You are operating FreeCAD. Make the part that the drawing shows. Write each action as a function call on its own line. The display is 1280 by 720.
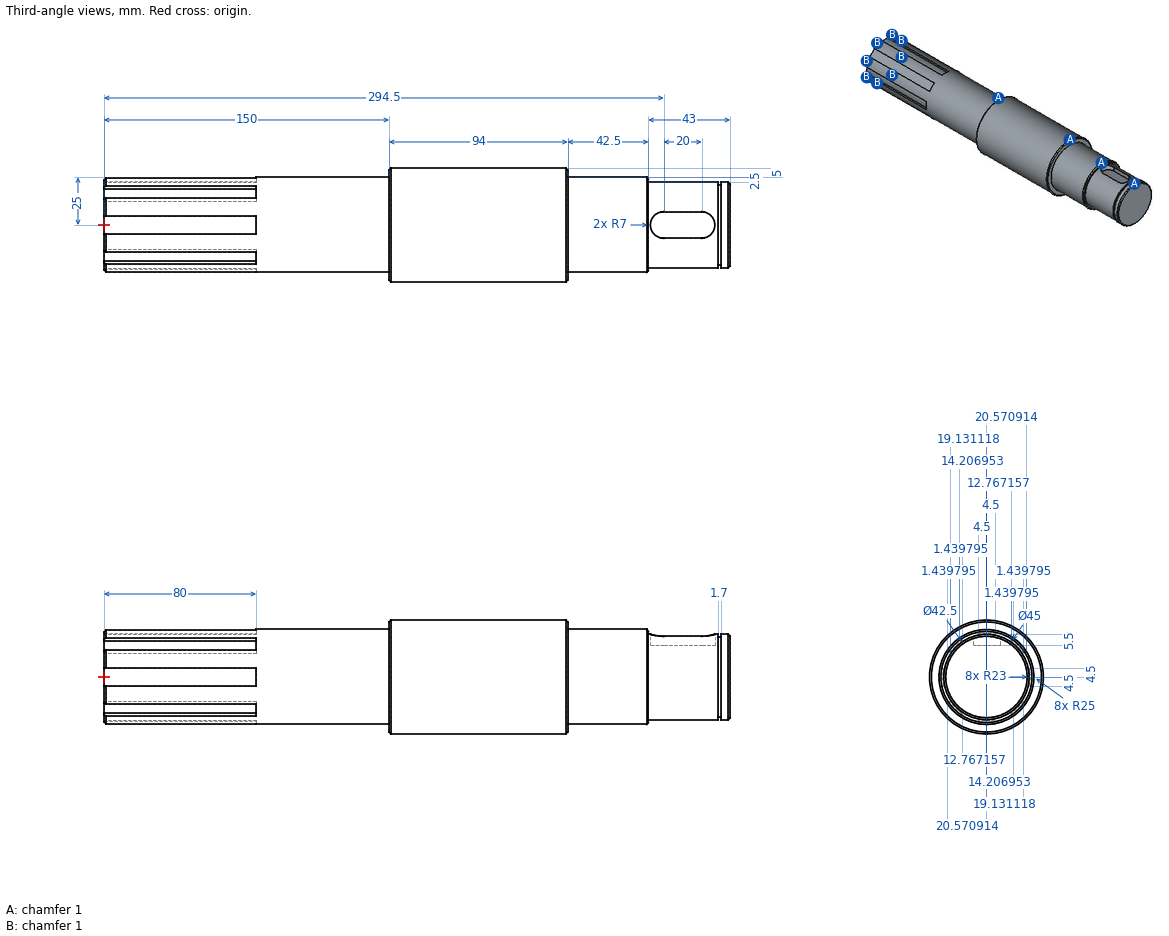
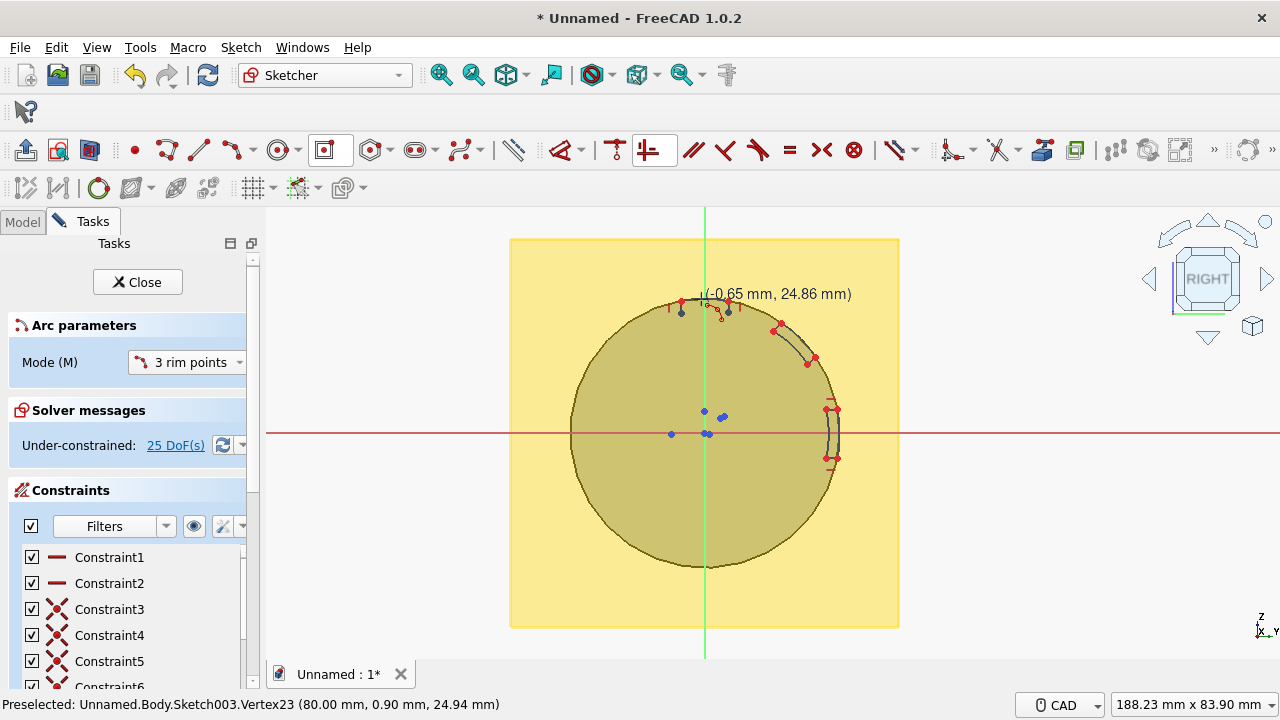
scroll(729, 312, up, 6)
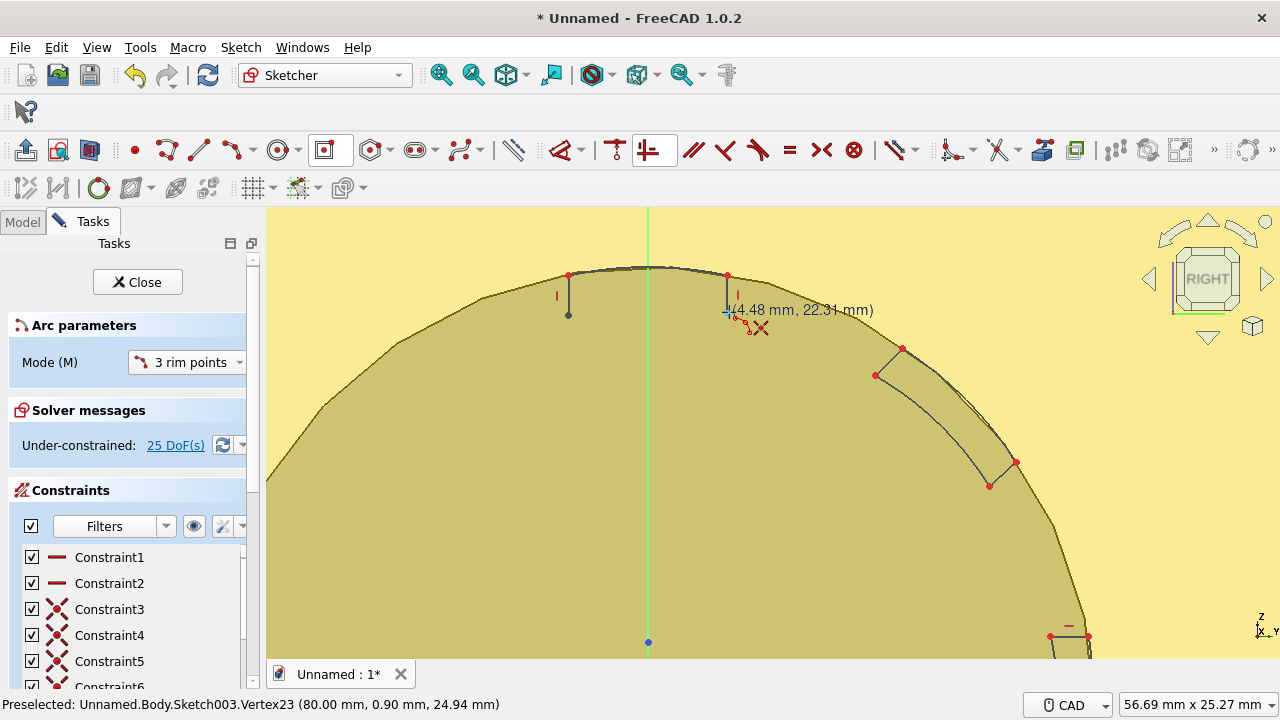
click(727, 313)
click(569, 315)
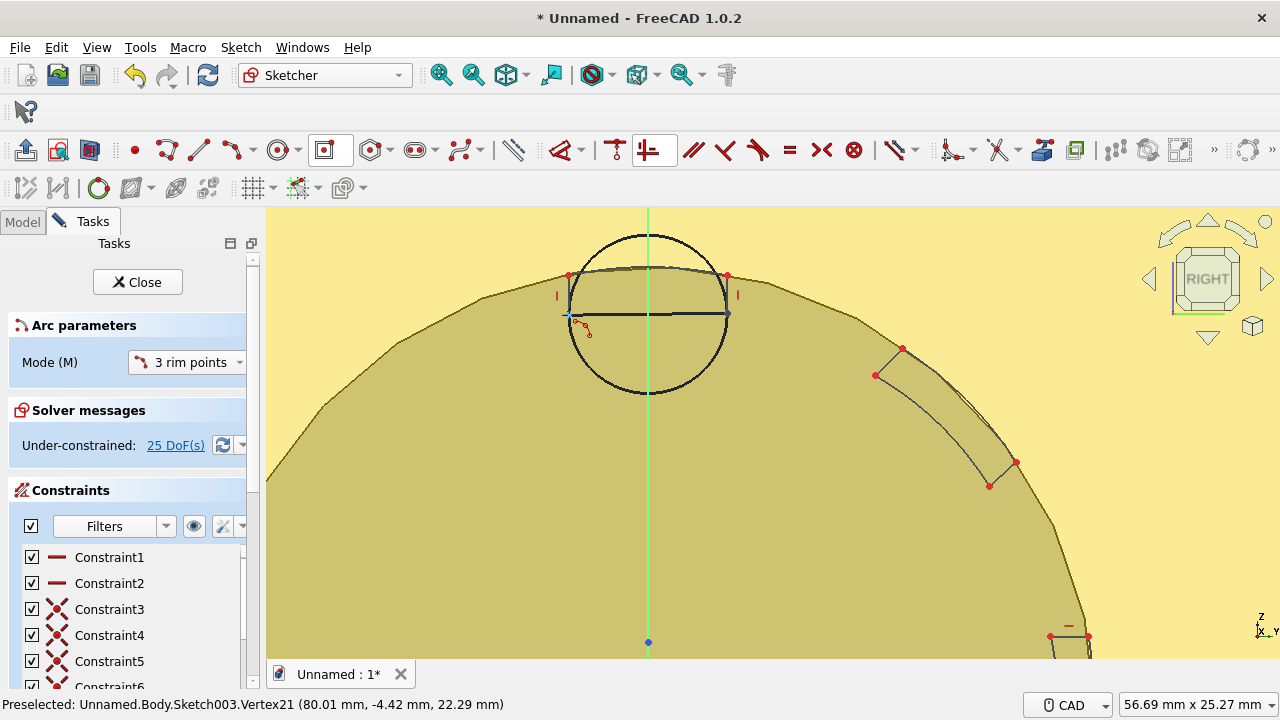
scroll(664, 303, up, 4)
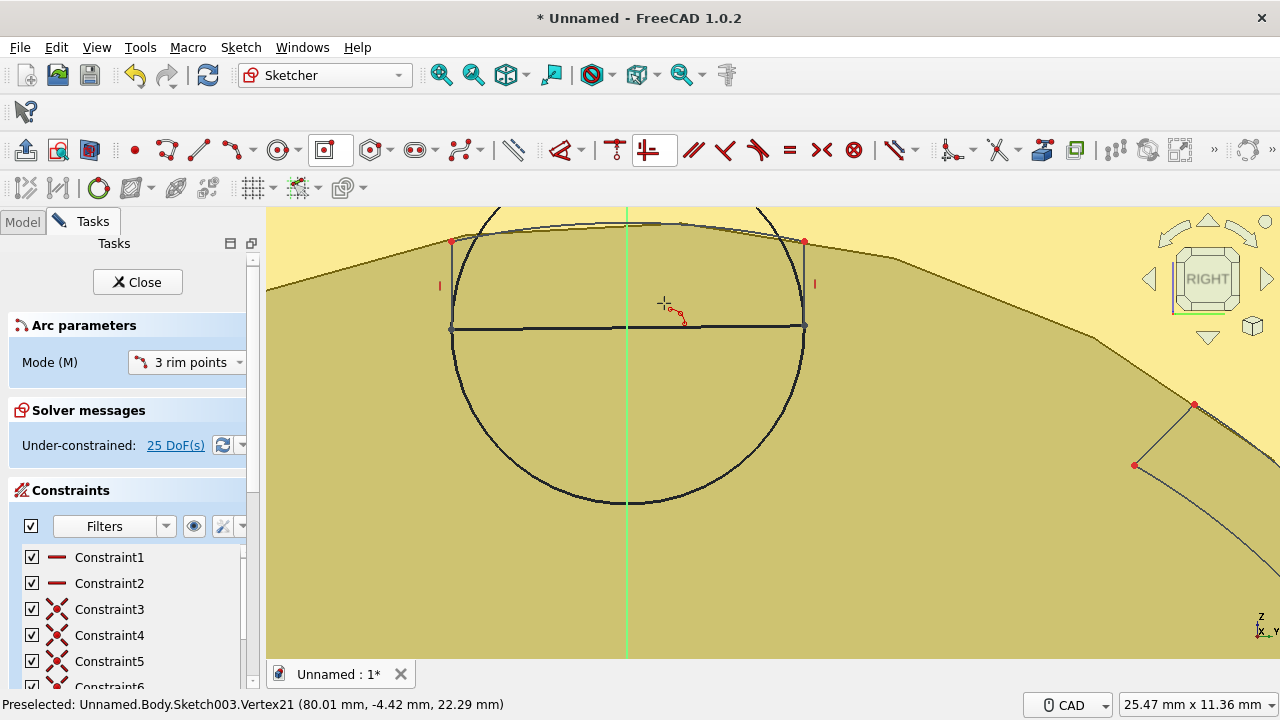
click(664, 302)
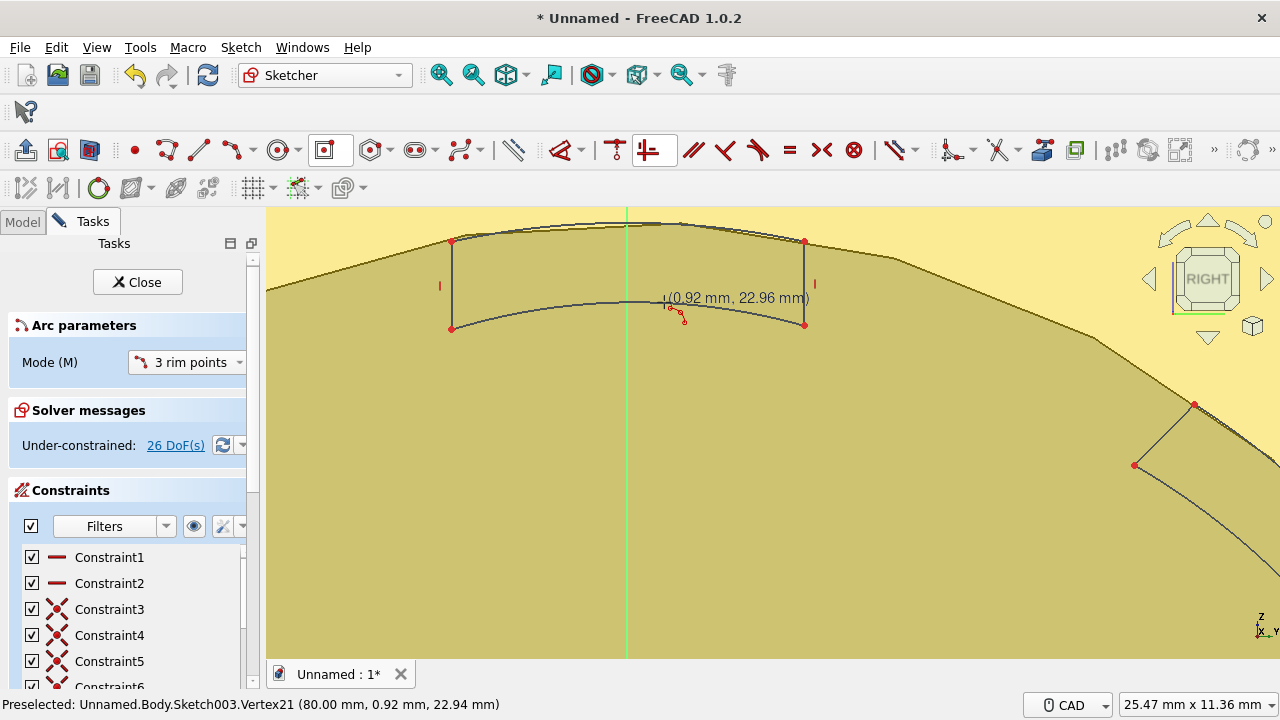
click(200, 150)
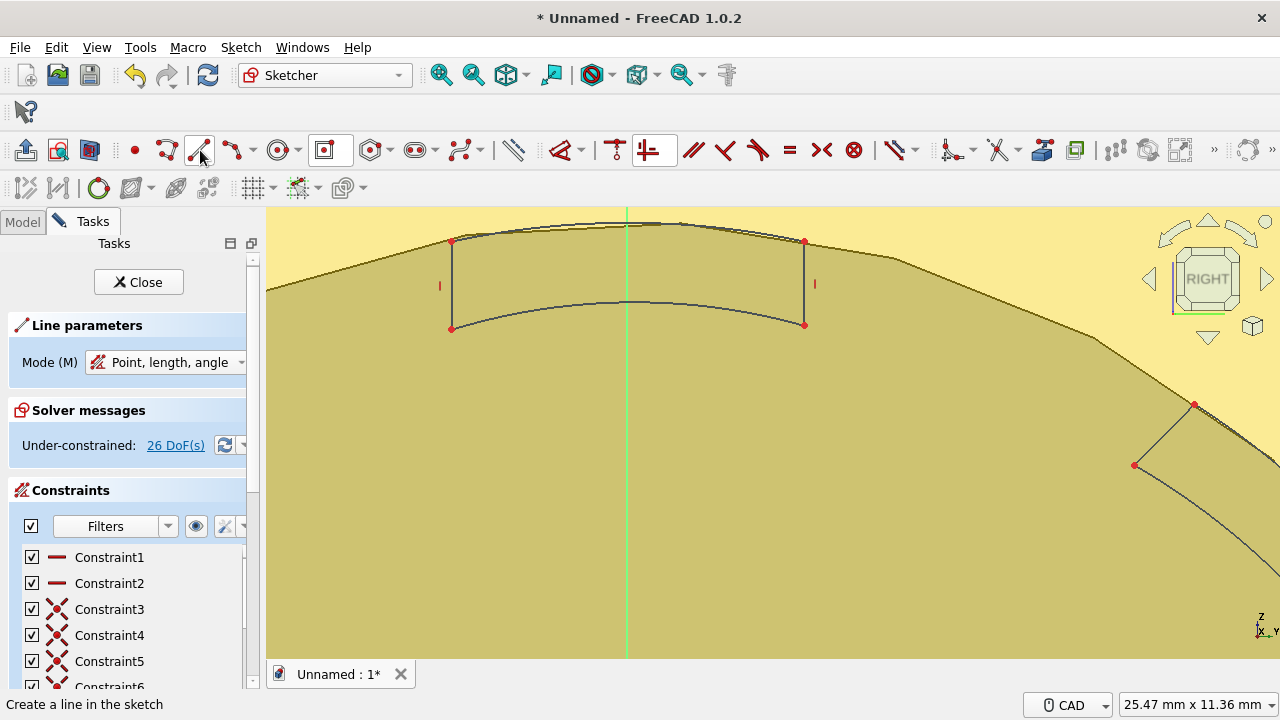
scroll(717, 310, down, 10)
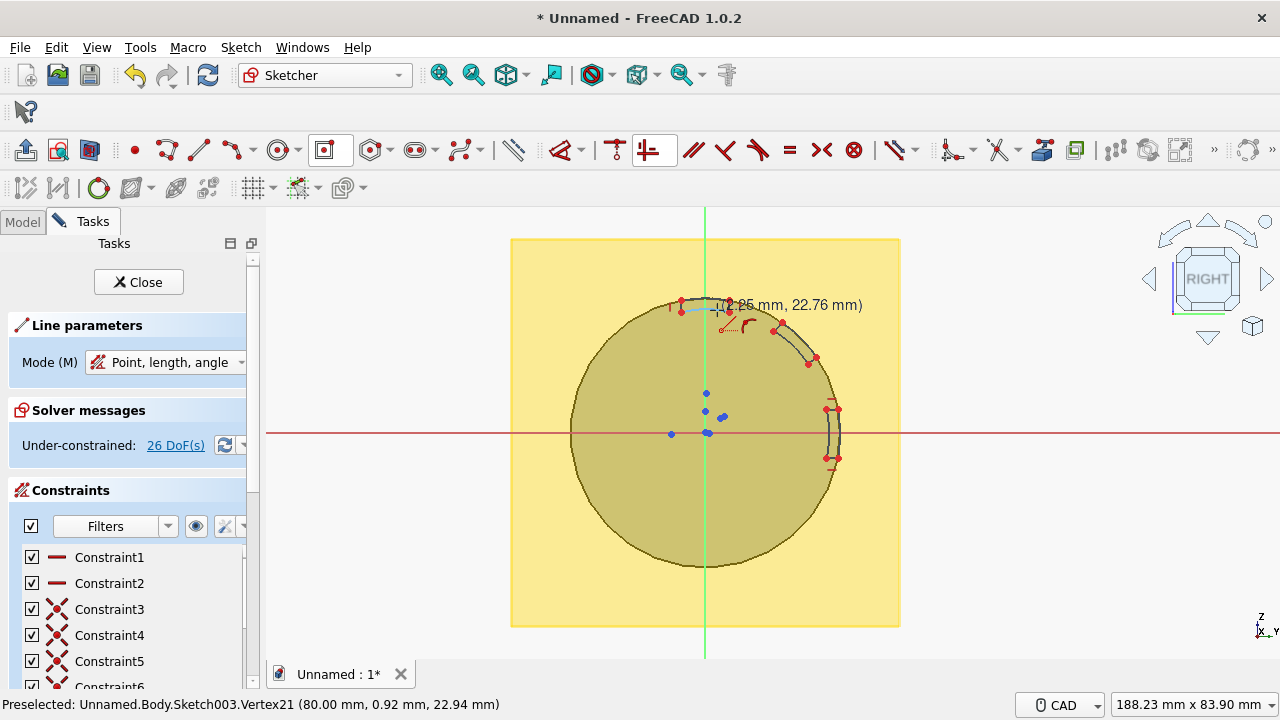
click(602, 364)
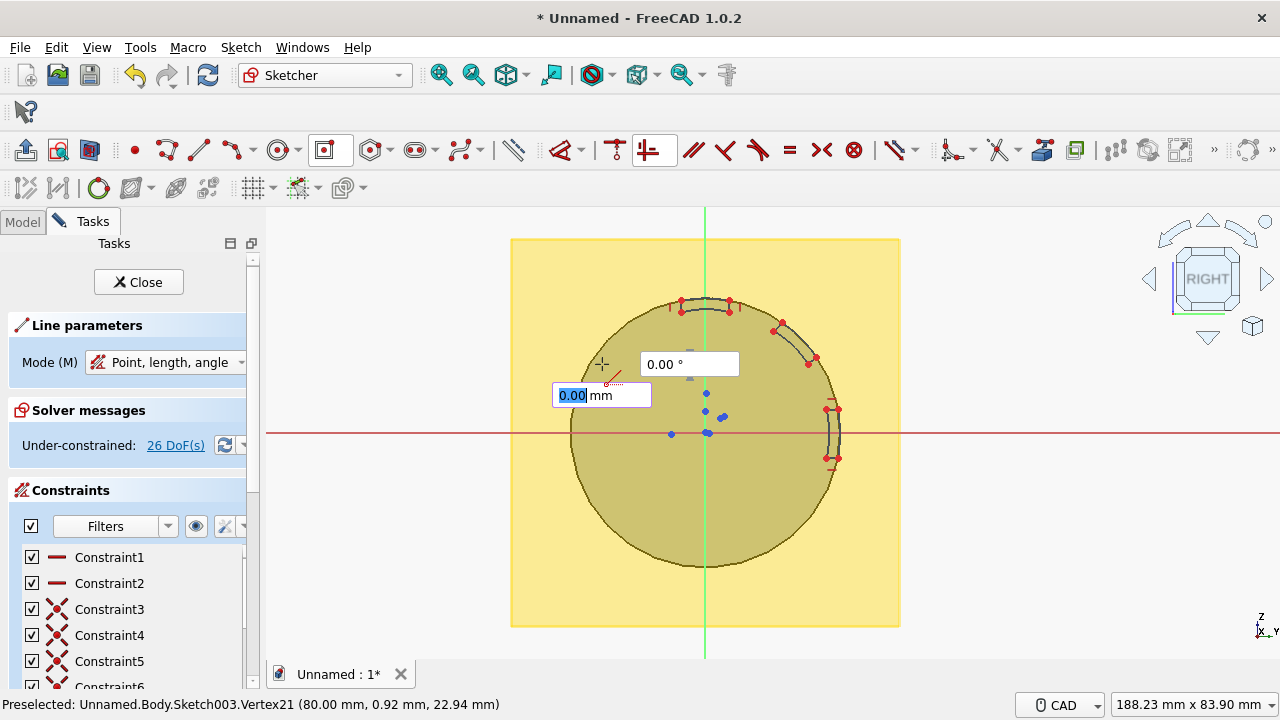
scroll(594, 356, up, 2)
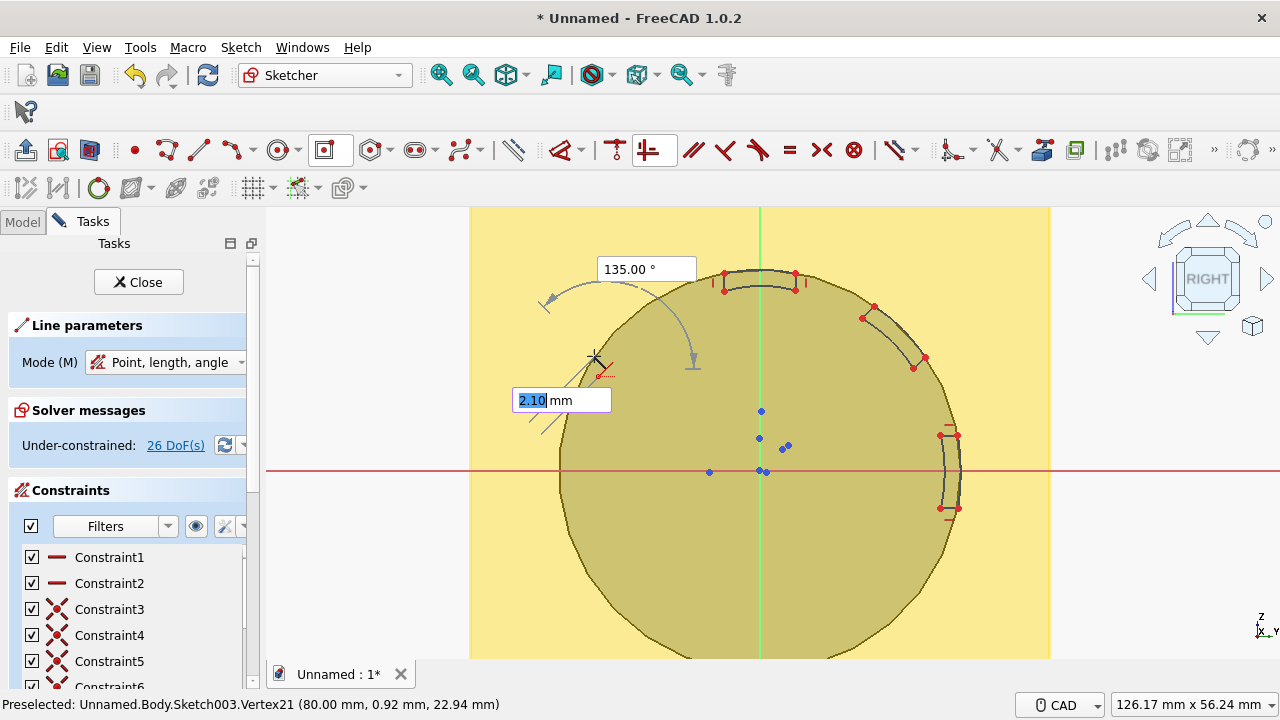
click(595, 356)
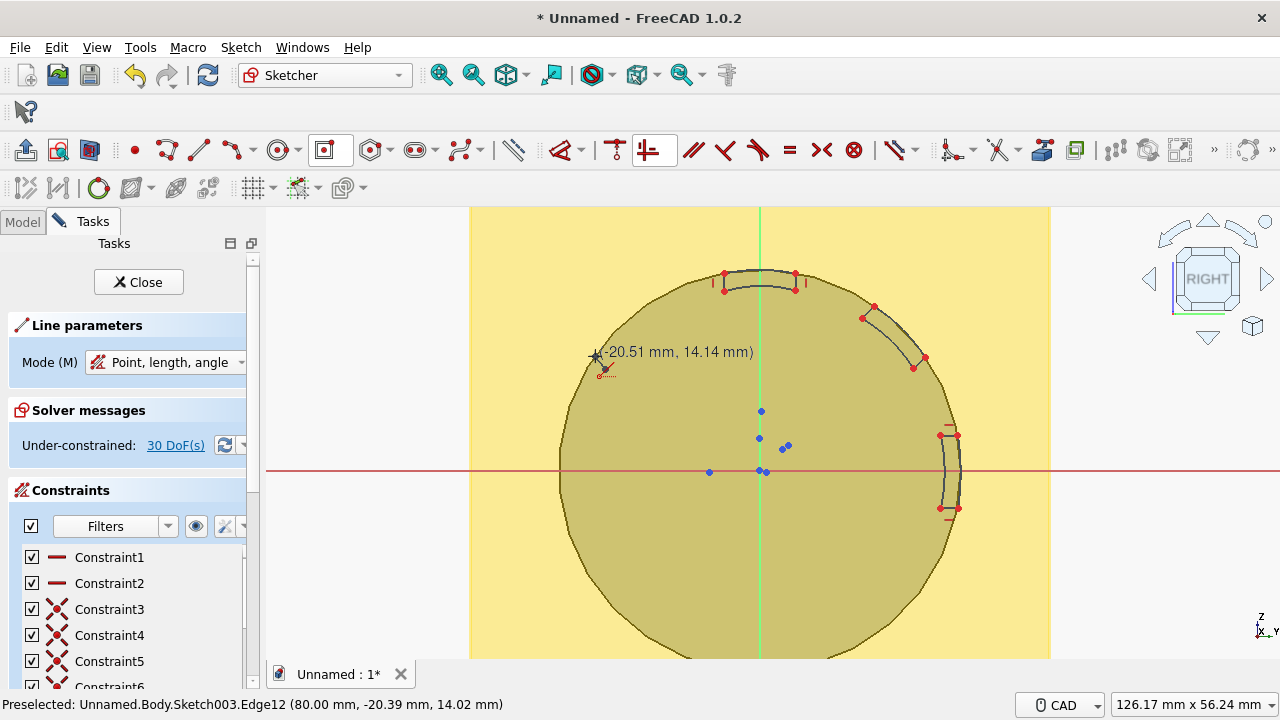
click(646, 305)
click(657, 317)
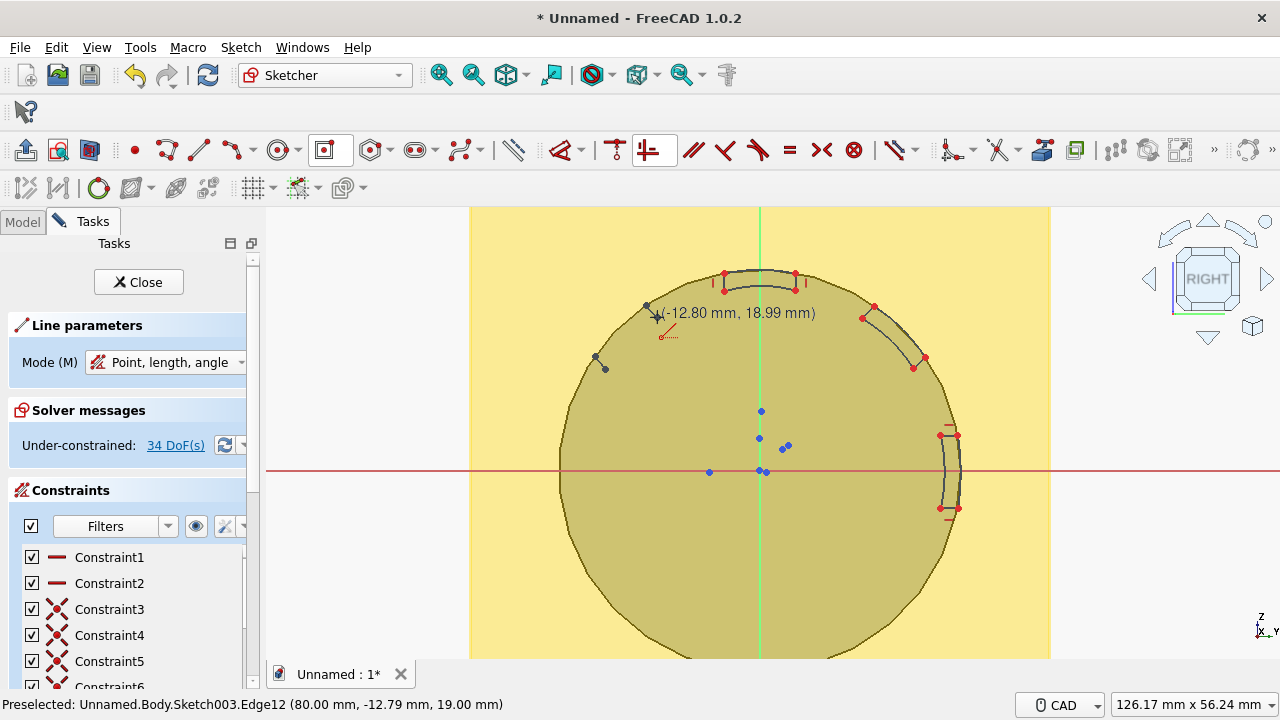
click(232, 150)